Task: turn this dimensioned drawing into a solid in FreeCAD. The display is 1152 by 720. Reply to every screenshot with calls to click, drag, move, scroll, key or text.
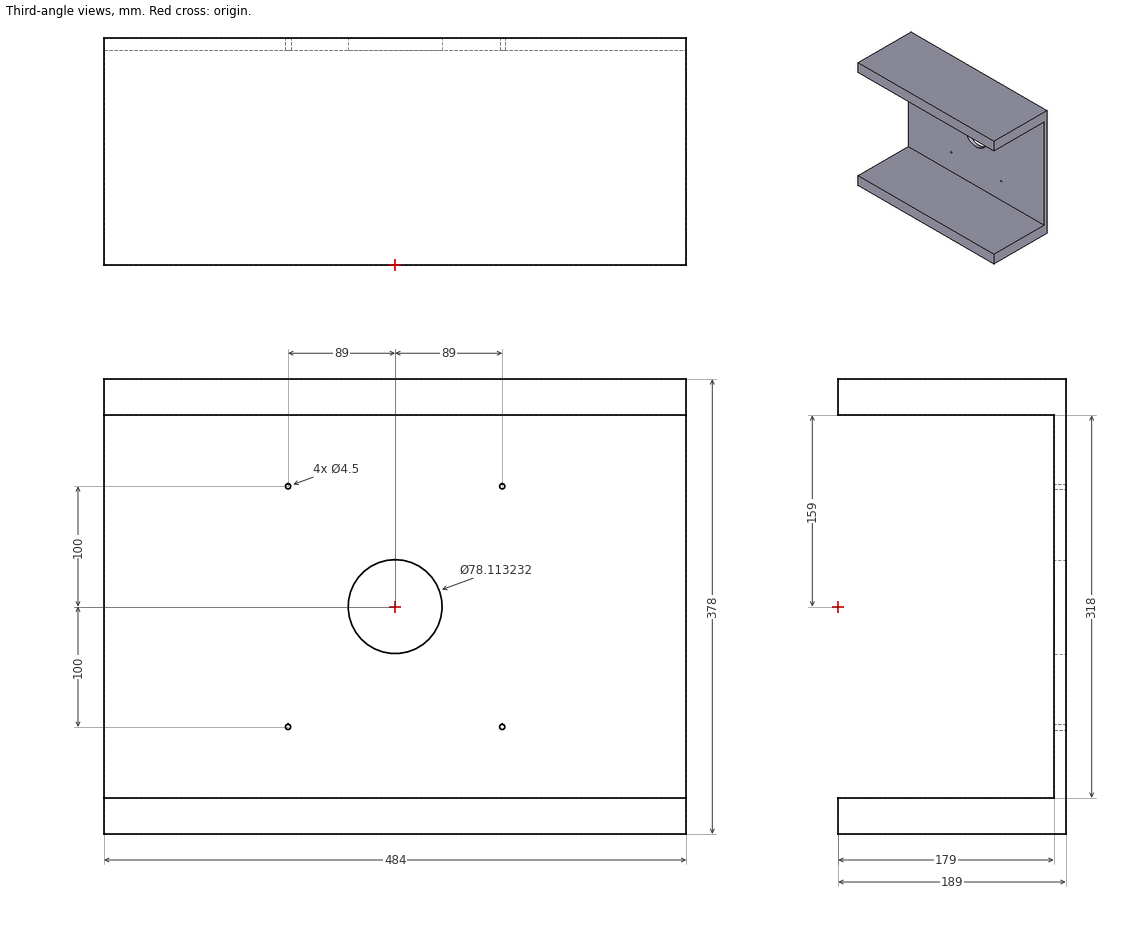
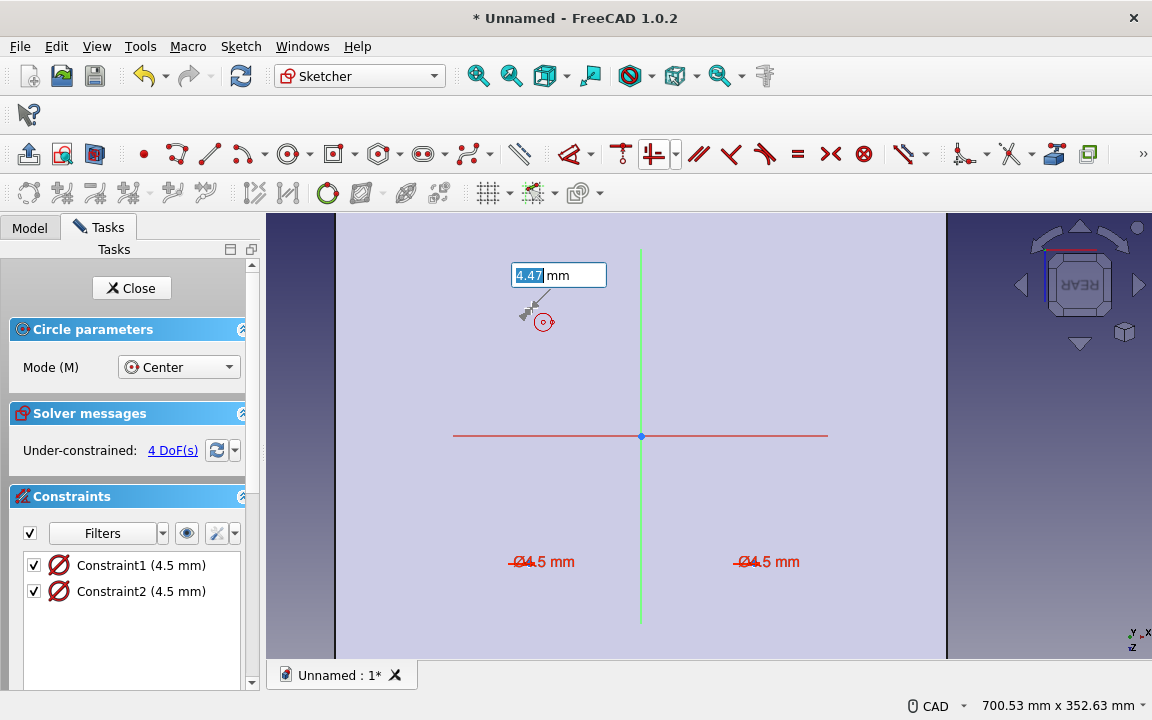
text(4.5)
key(Return)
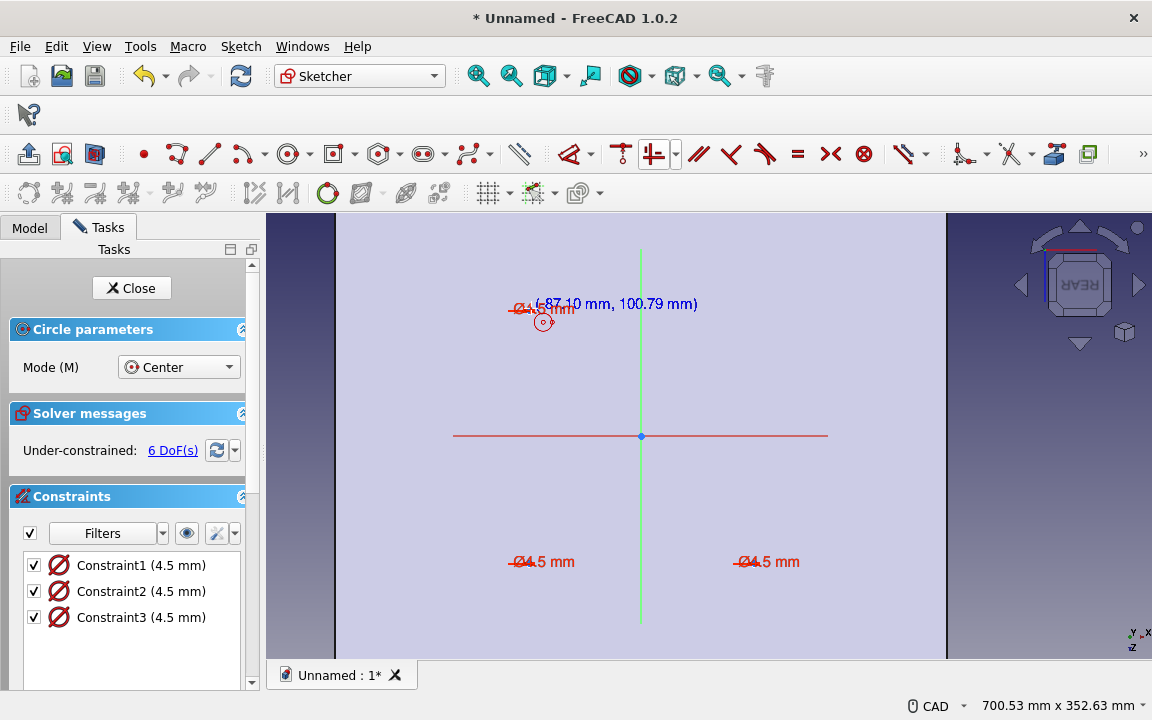
scroll(754, 310, up, 11)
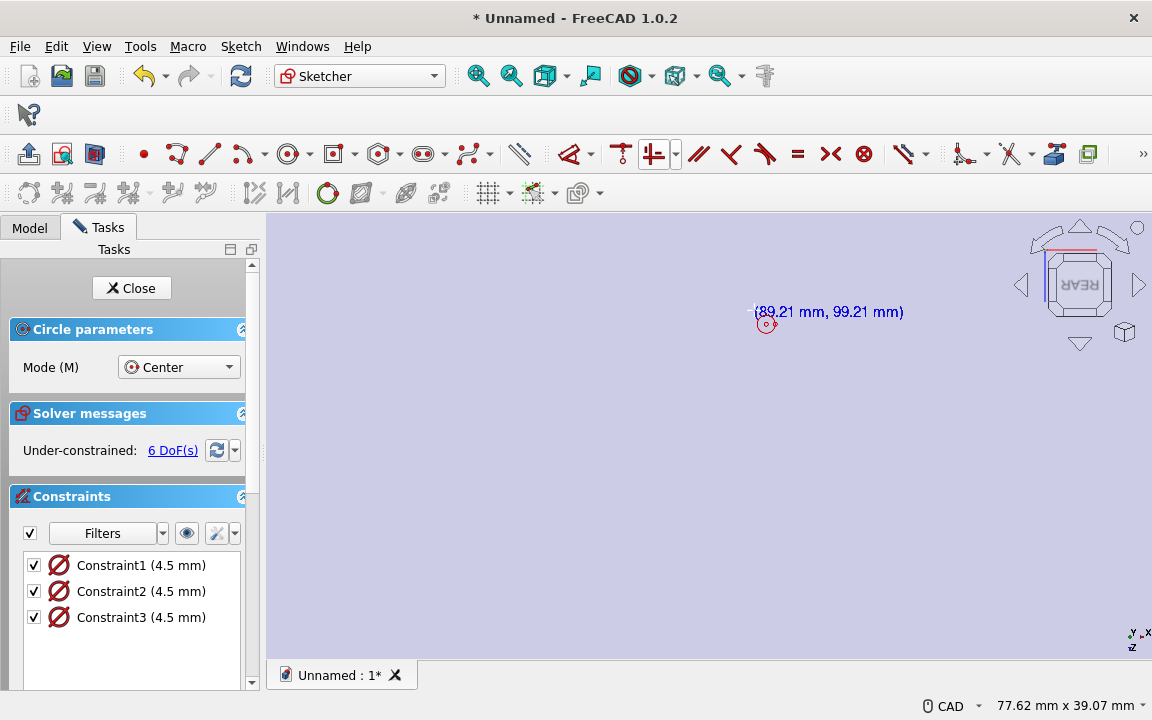
scroll(754, 310, down, 11)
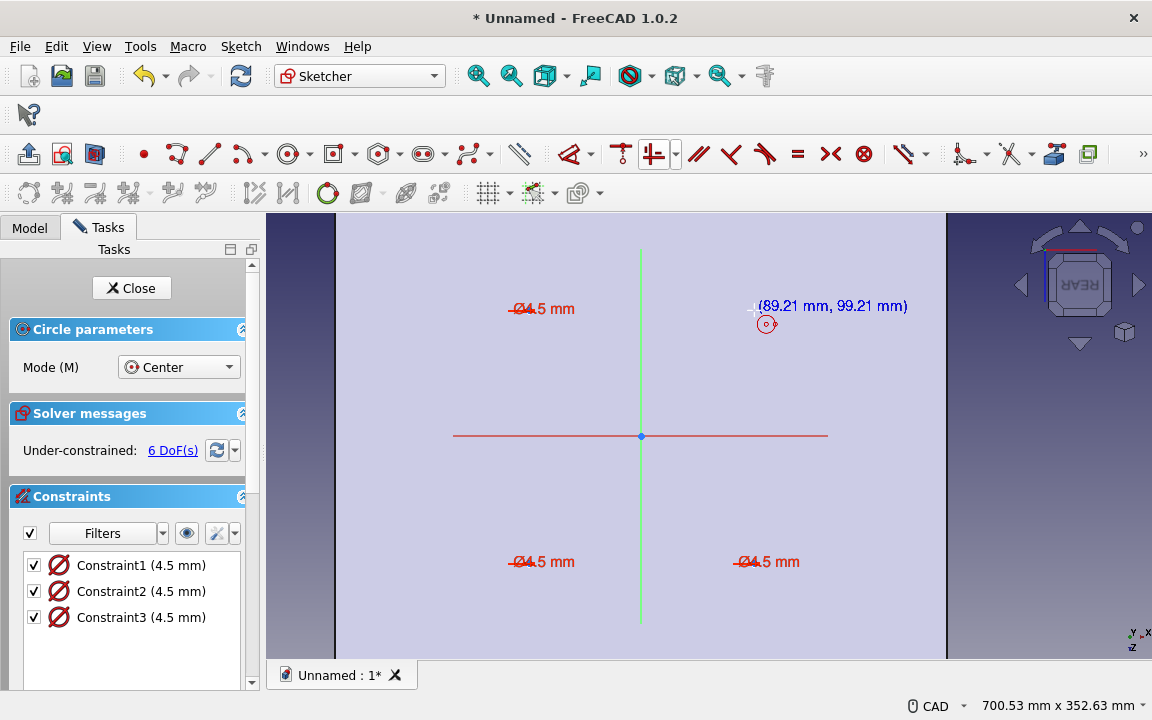
click(754, 310)
move(756, 308)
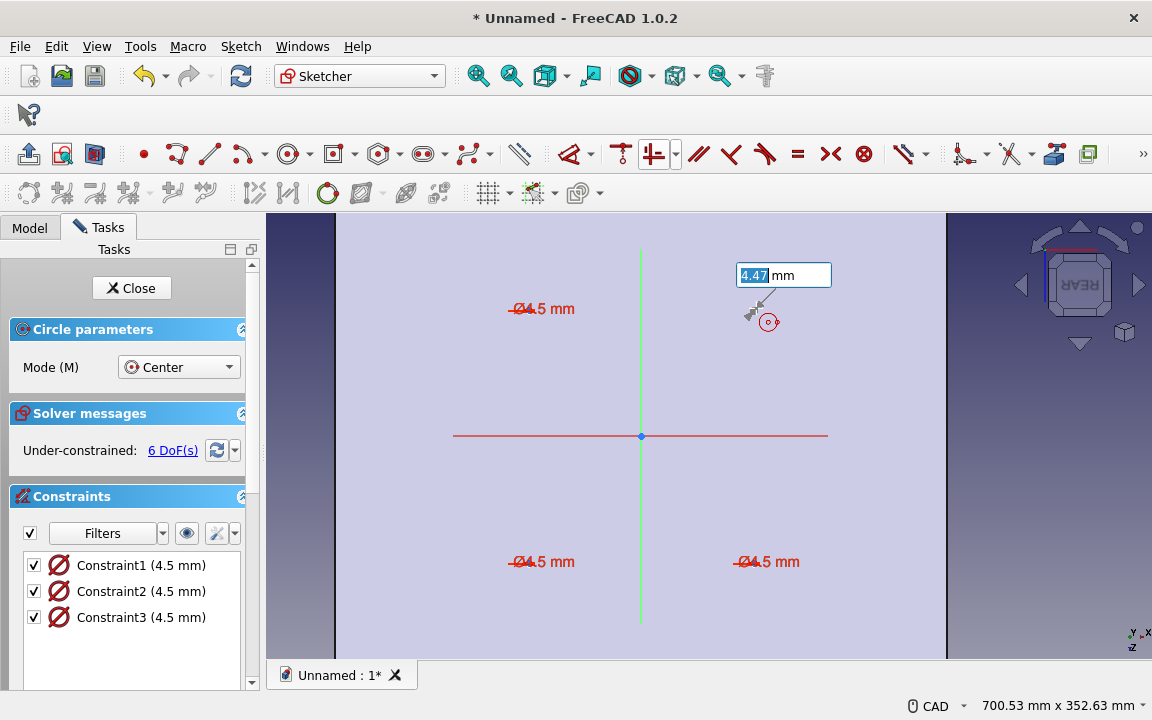
text(4.5)
key(Return)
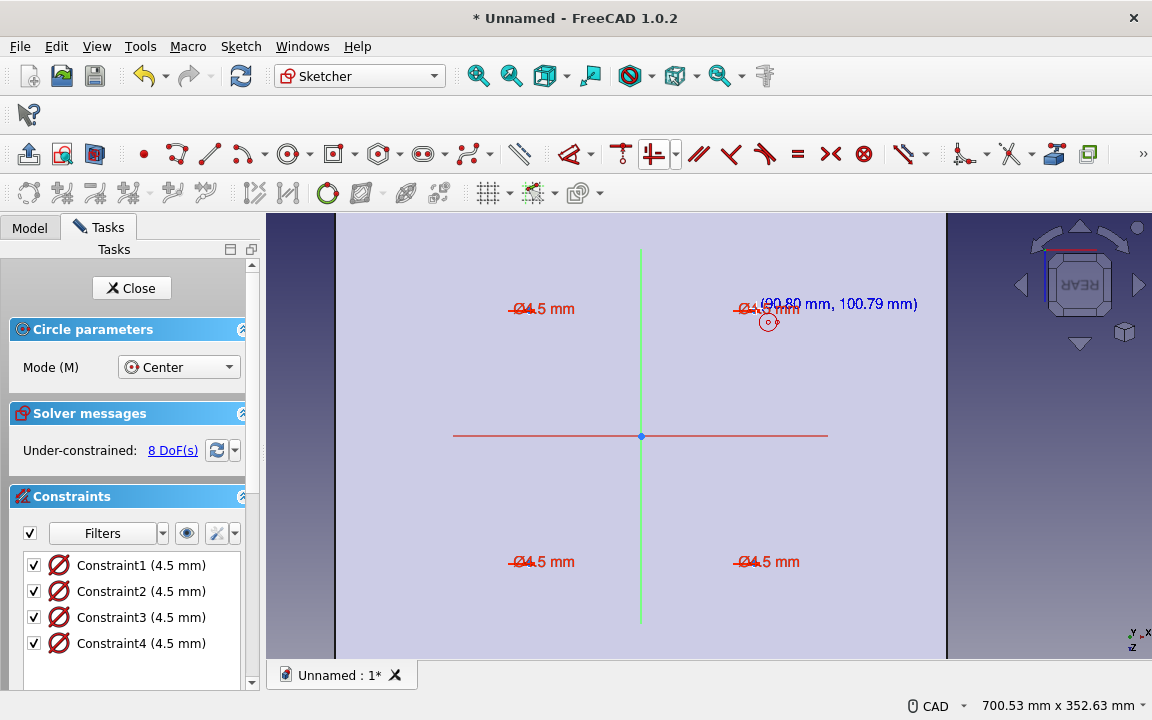
click(641, 436)
move(676, 402)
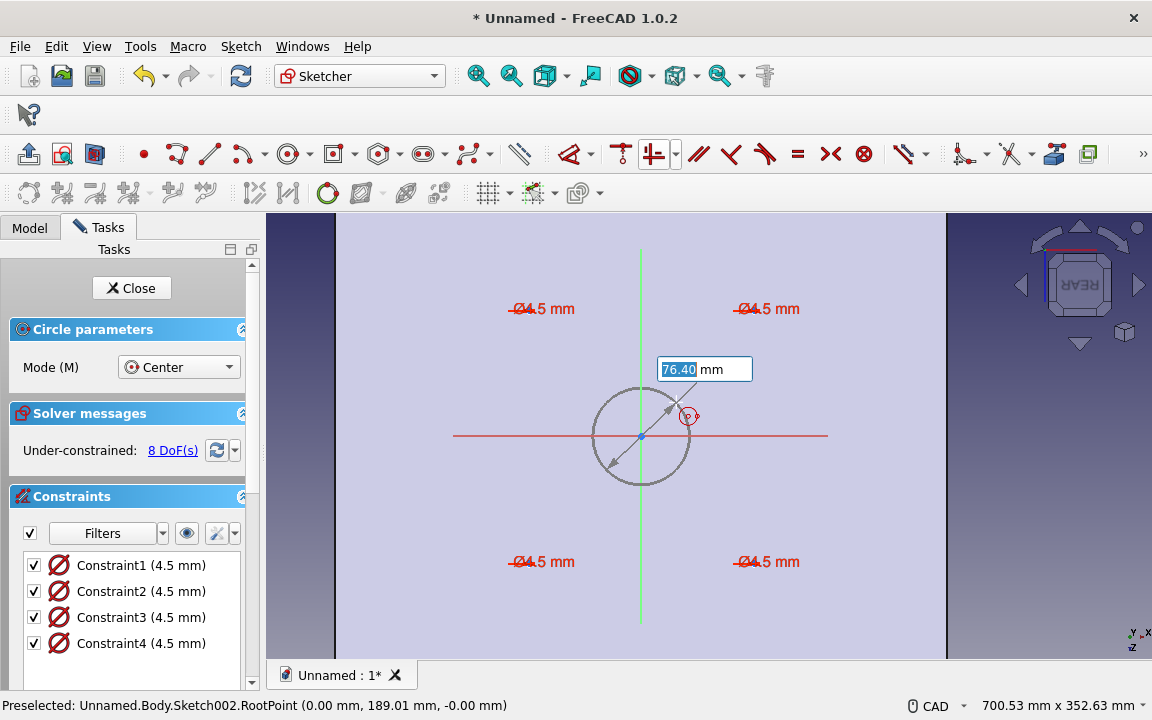
text(78.113232)
key(Return)
key(Escape)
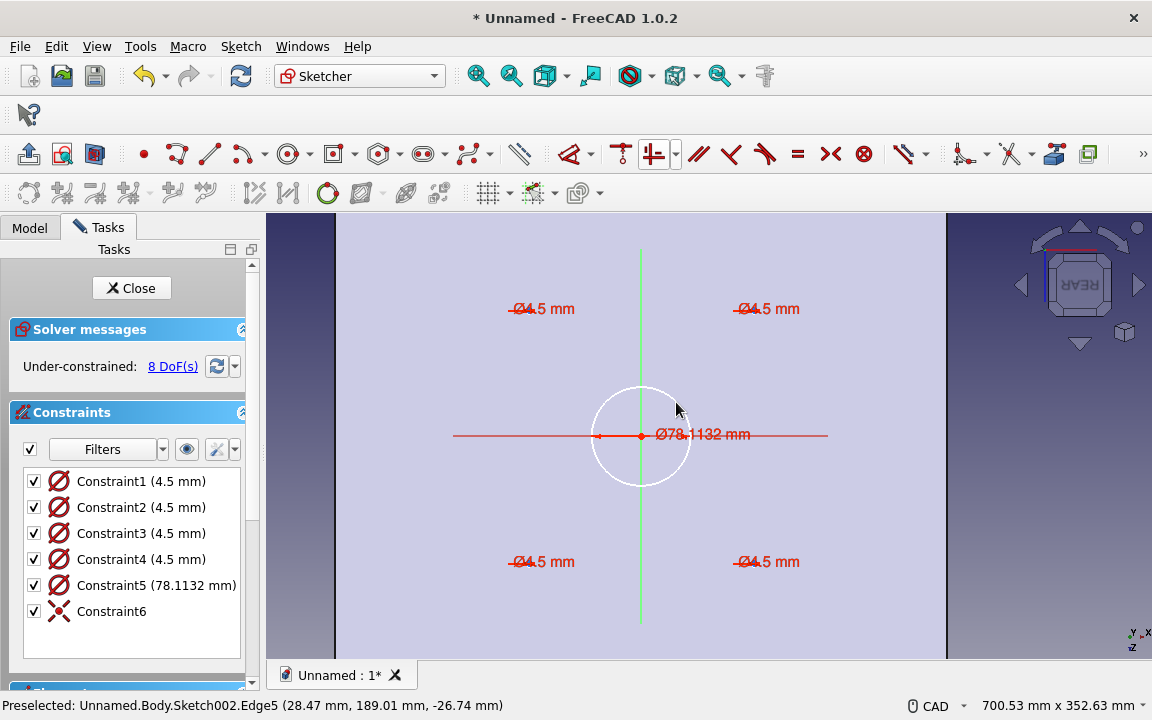
click(529, 564)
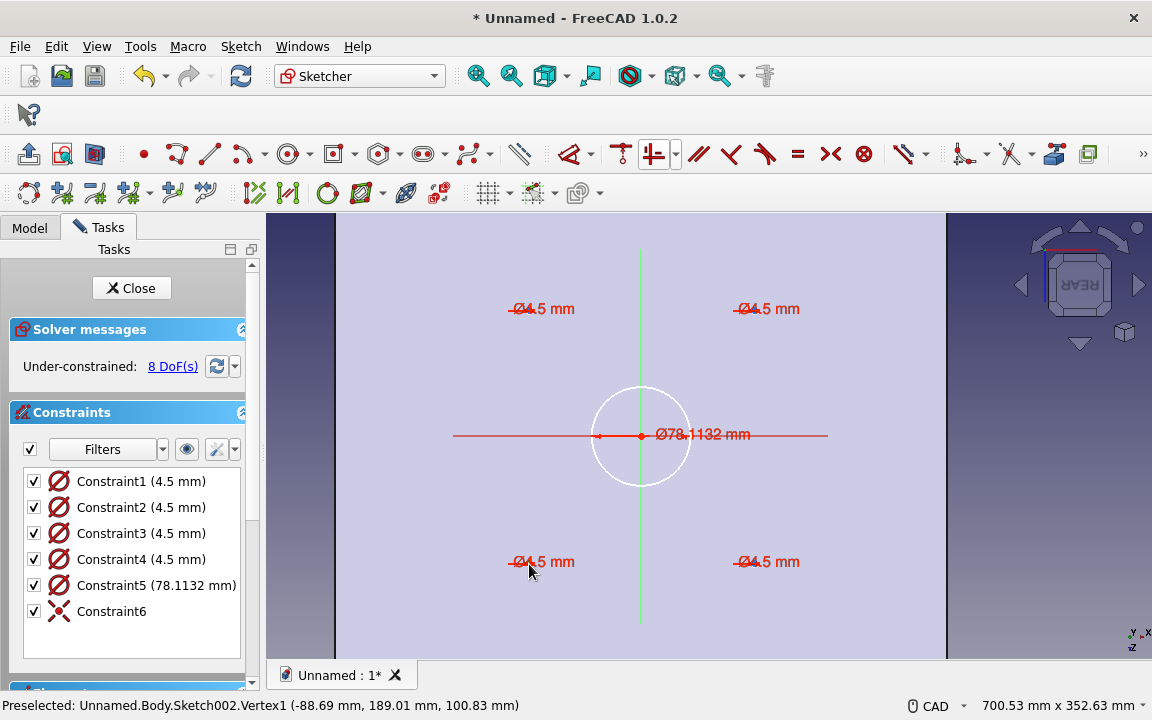
click(754, 564)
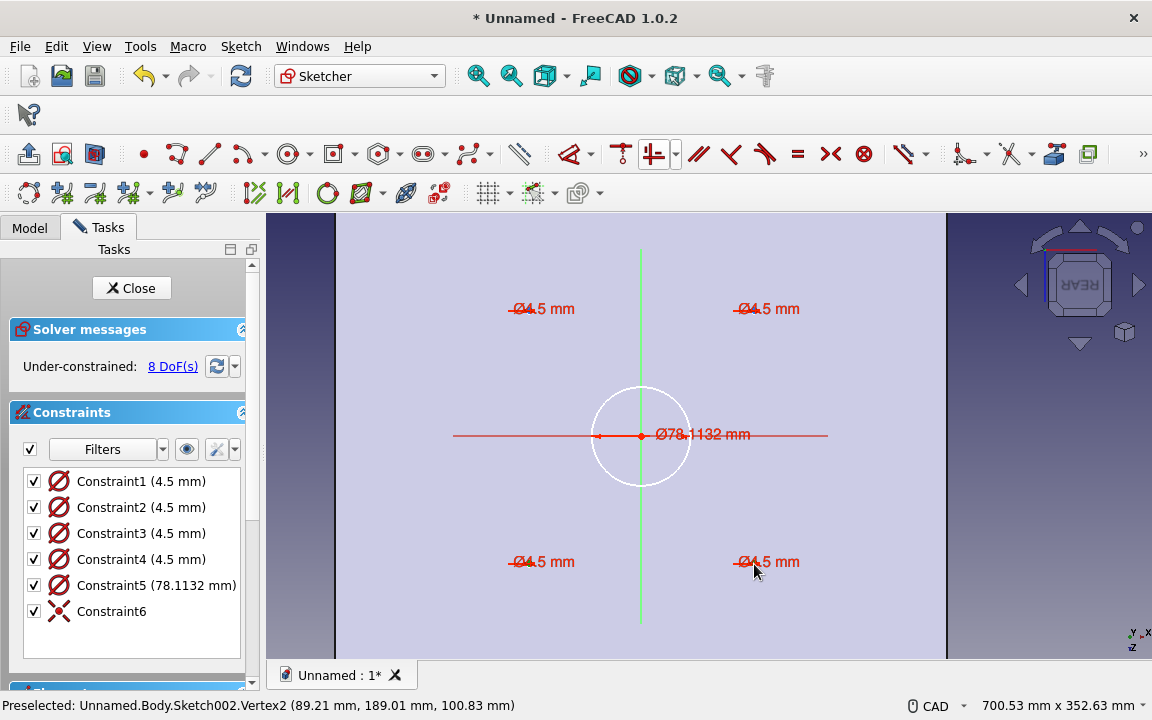
click(676, 154)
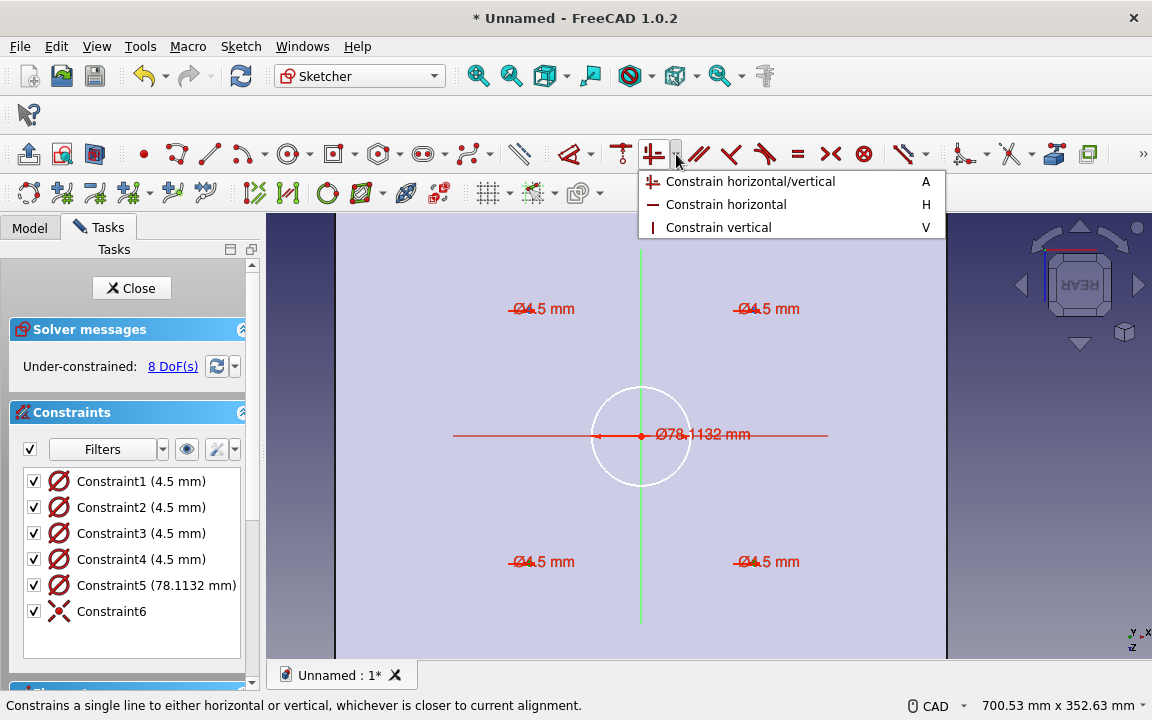
click(792, 204)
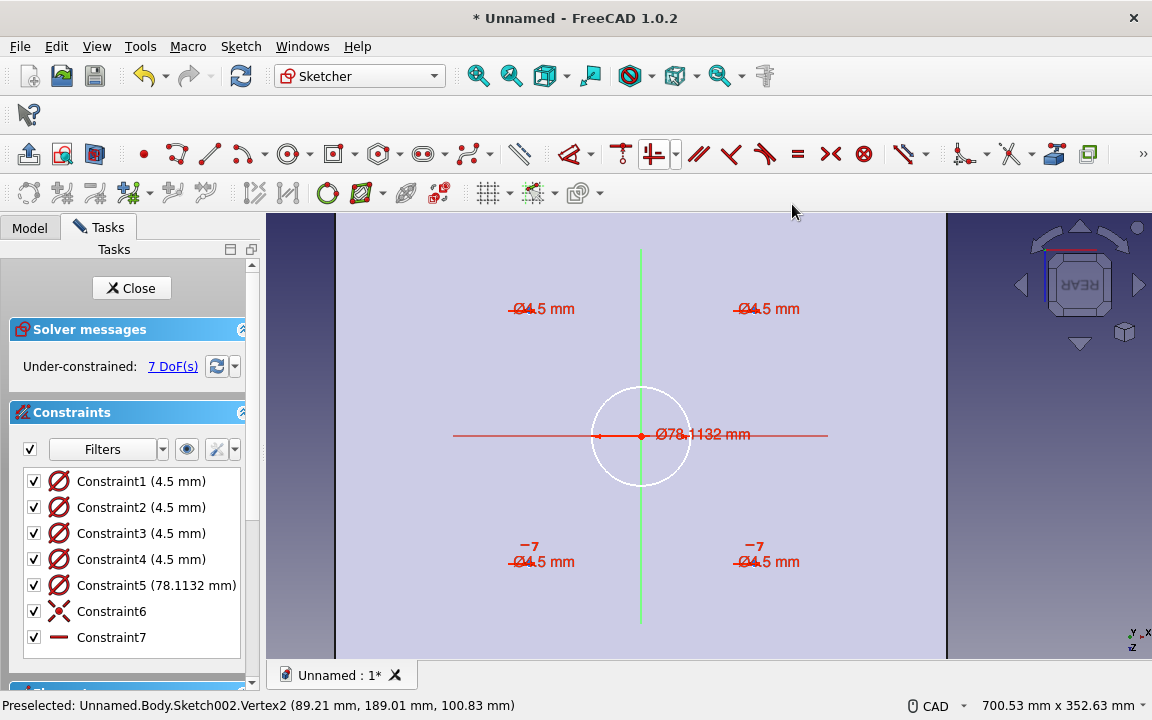
click(529, 564)